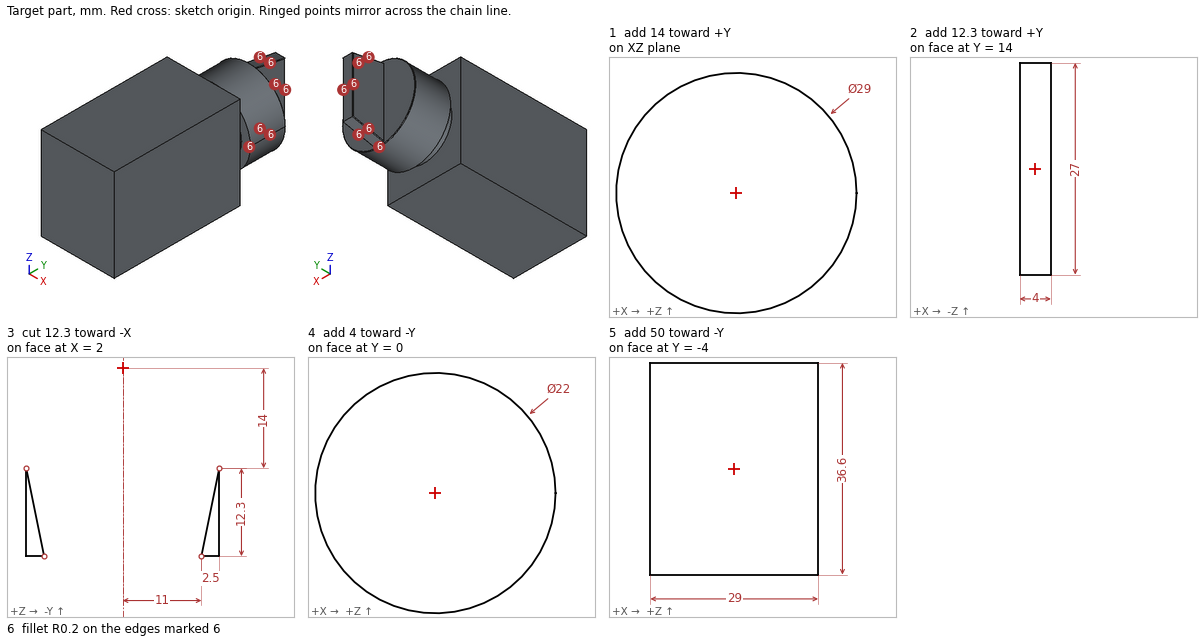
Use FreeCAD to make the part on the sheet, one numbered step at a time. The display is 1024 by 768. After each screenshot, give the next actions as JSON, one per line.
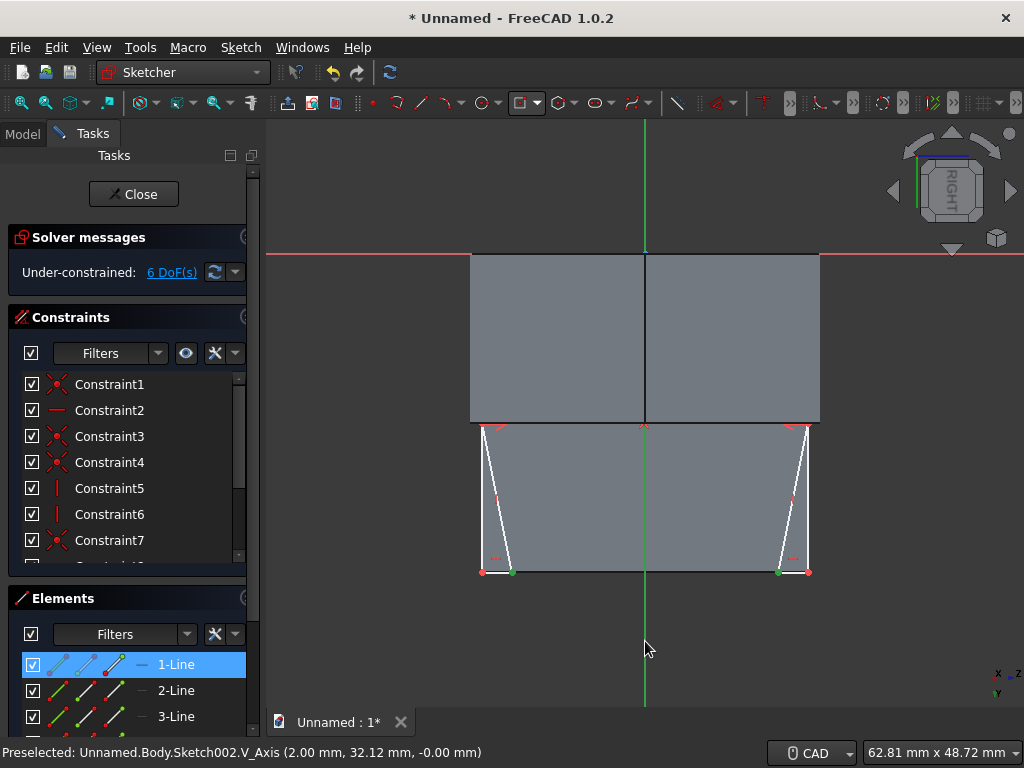
{"action": "key", "text": "s"}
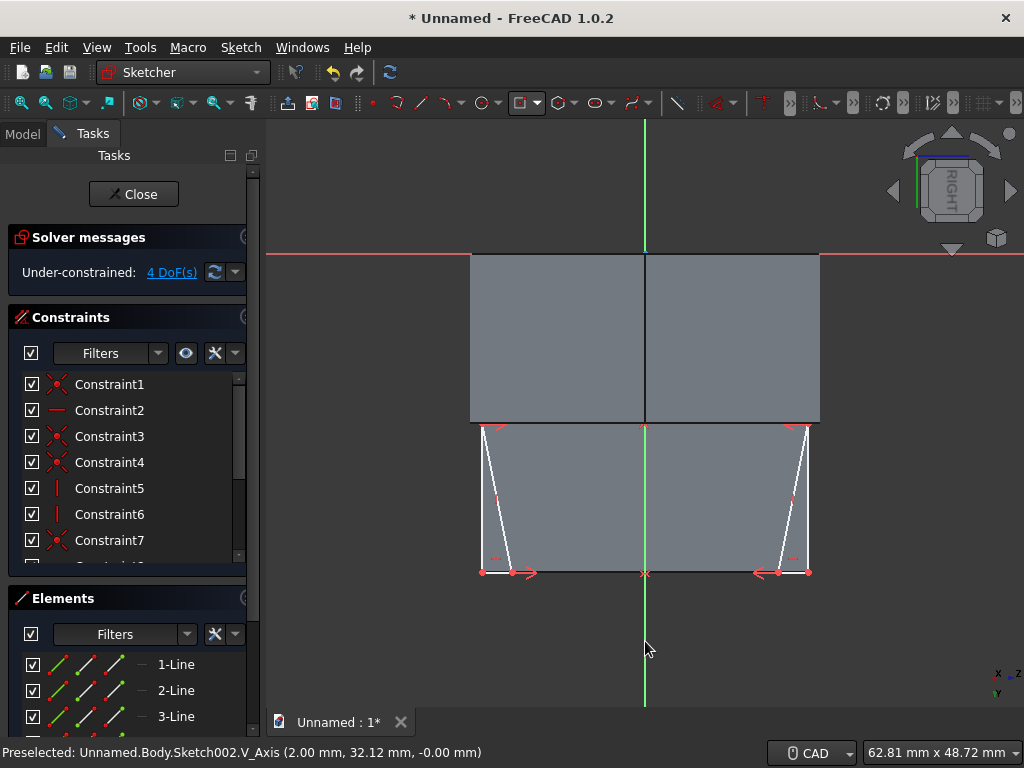
{"action": "left_click", "coordinate": [716, 104]}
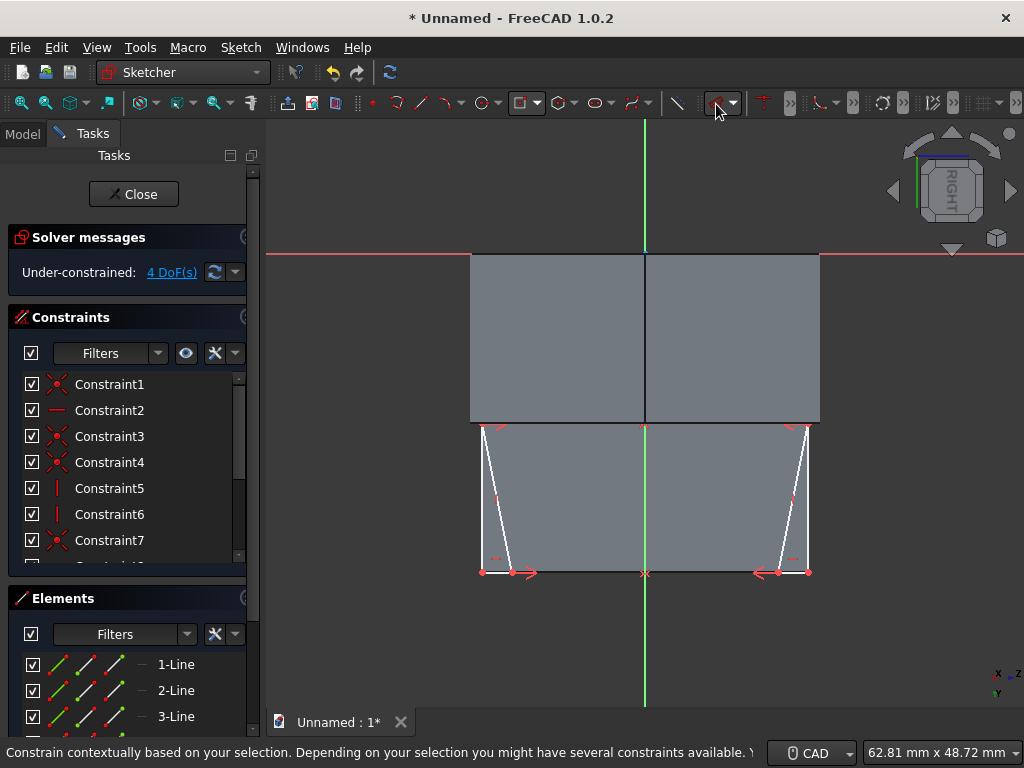
{"action": "scroll", "coordinate": [790, 573], "scroll_direction": "up", "scroll_amount": 2}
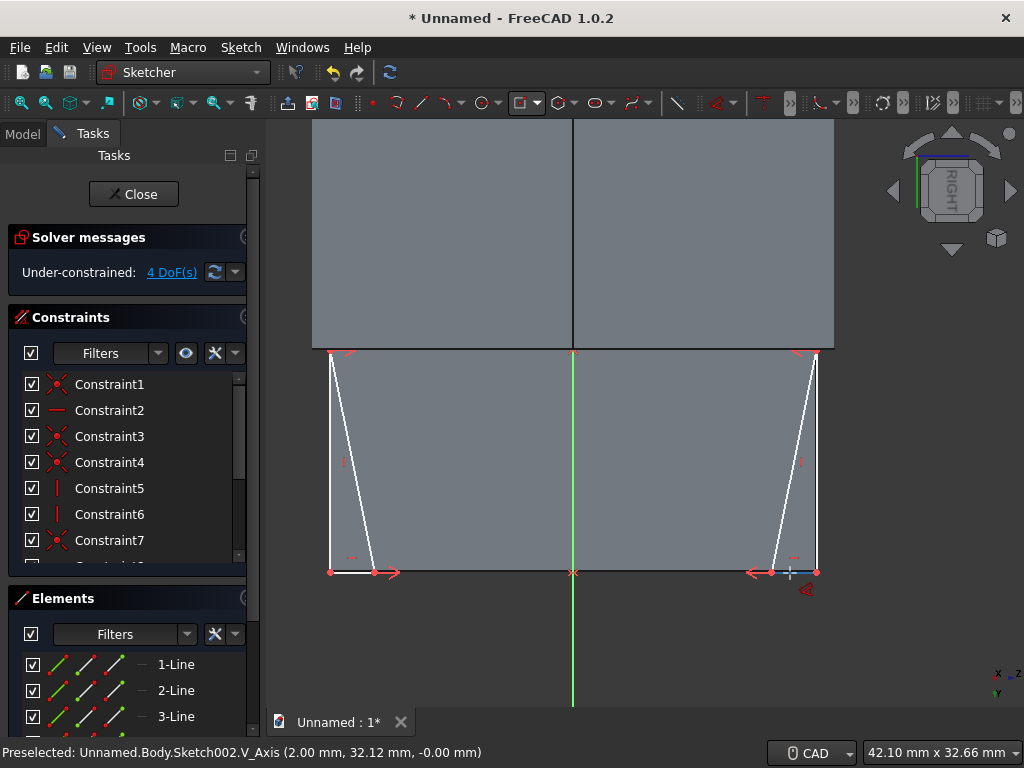
{"action": "left_click", "coordinate": [790, 573]}
{"action": "left_click", "coordinate": [794, 607]}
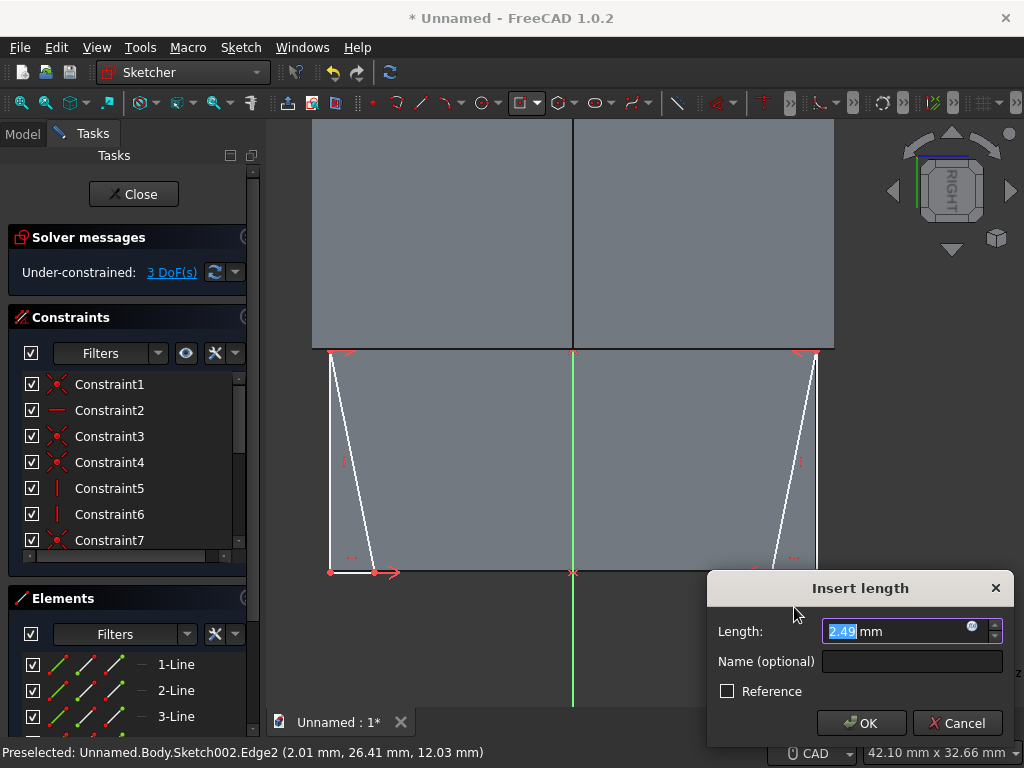
{"action": "type", "text": "2.5"}
{"action": "key", "text": "Return"}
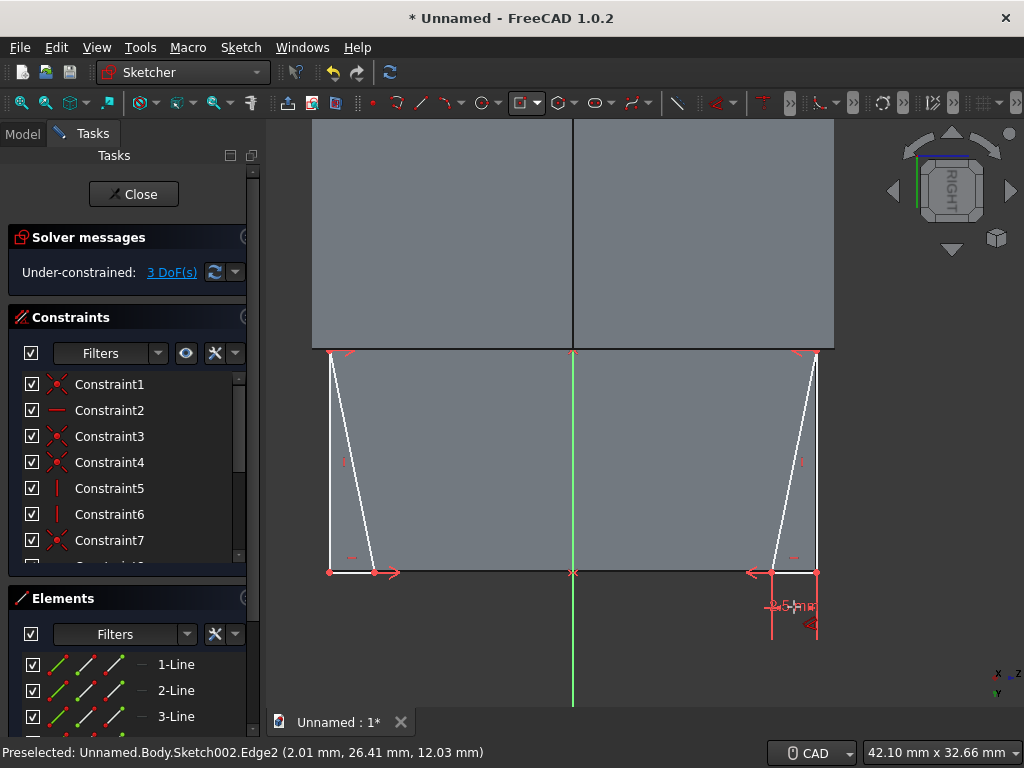
{"action": "left_click", "coordinate": [817, 350]}
{"action": "left_click", "coordinate": [851, 249]}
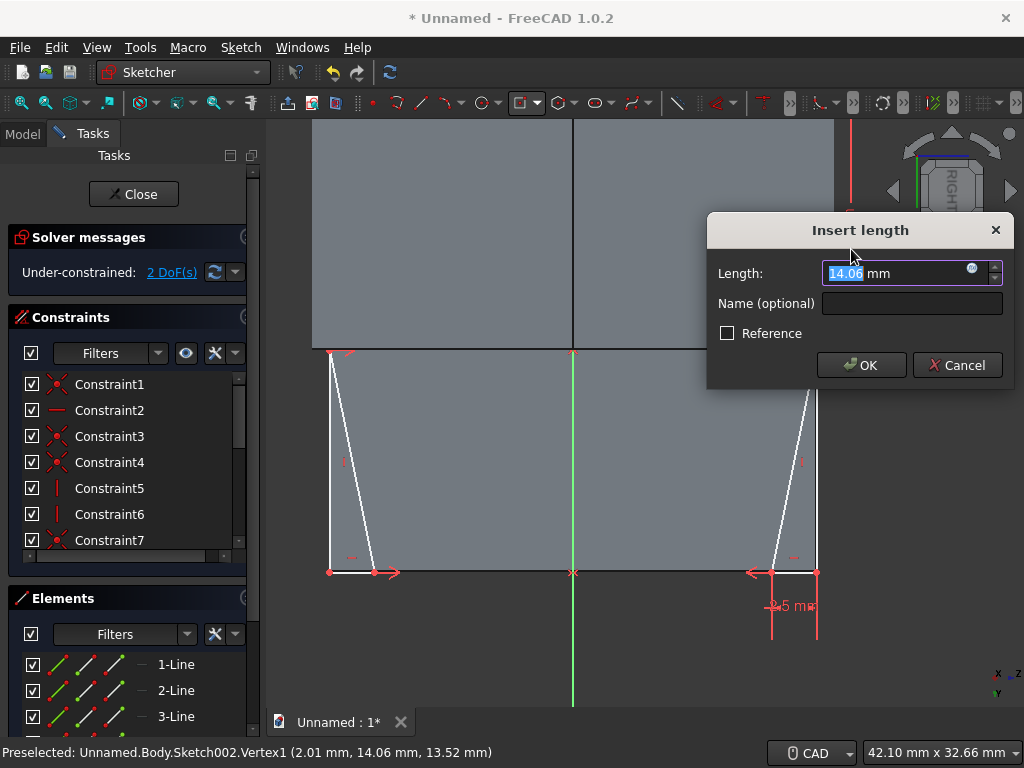
{"action": "type", "text": "14"}
{"action": "key", "text": "Return"}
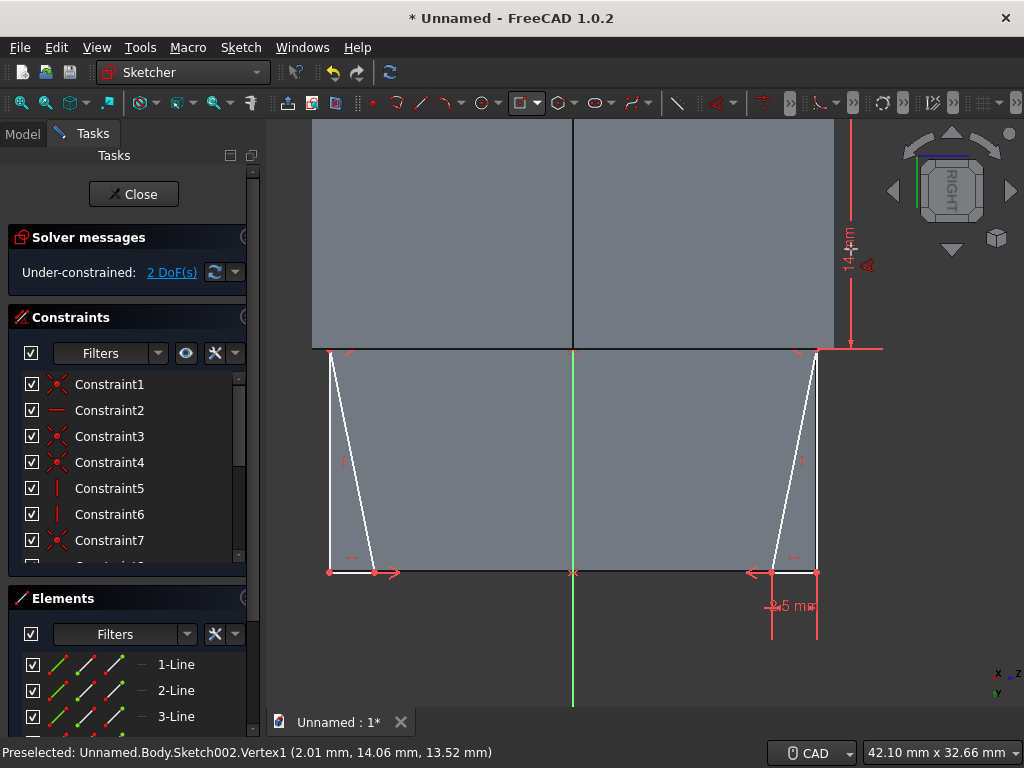
{"action": "left_click", "coordinate": [772, 573]}
{"action": "left_click", "coordinate": [673, 607]}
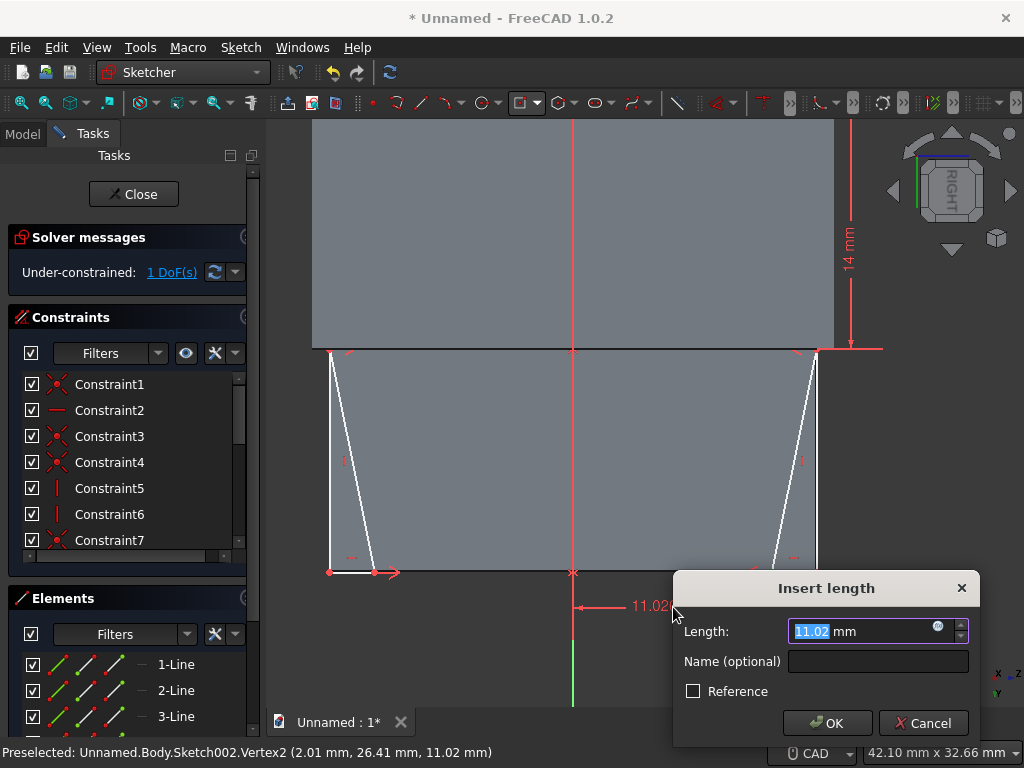
{"action": "type", "text": "11"}
{"action": "key", "text": "Return"}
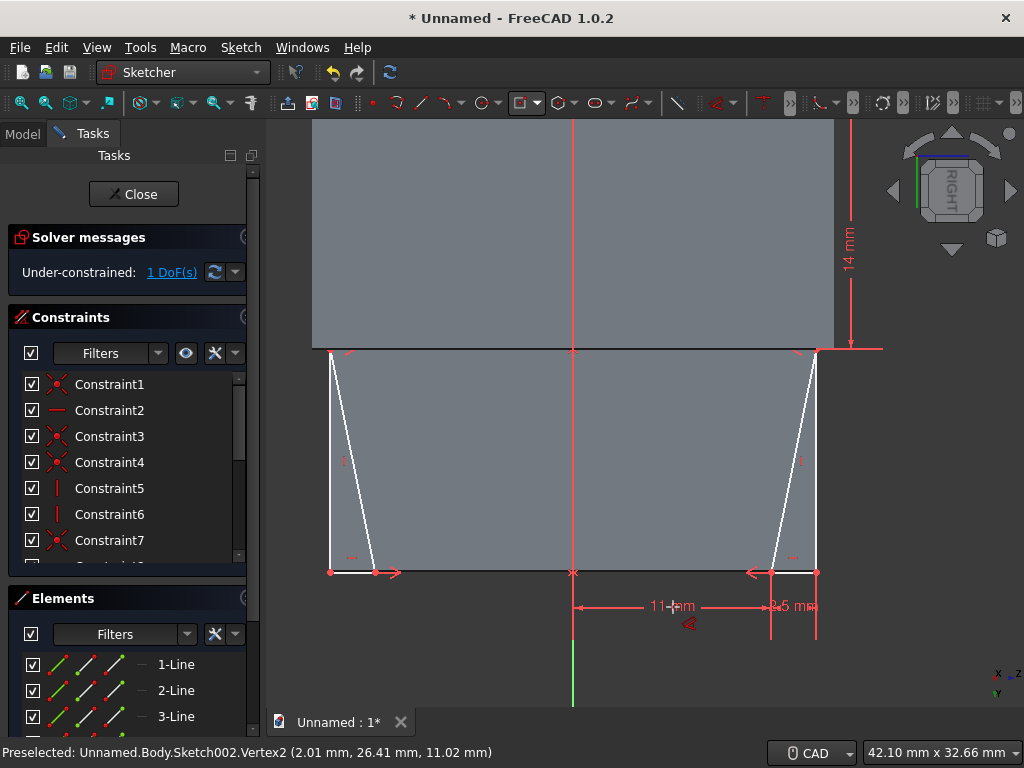
{"action": "left_click", "coordinate": [816, 506]}
{"action": "left_click", "coordinate": [850, 461]}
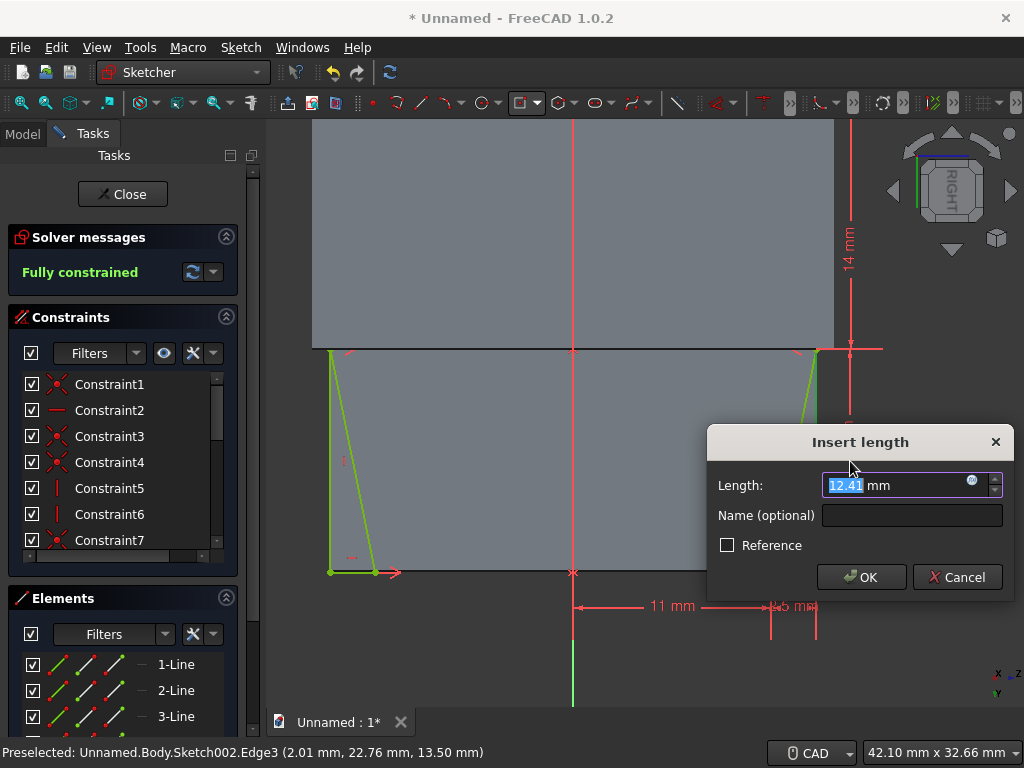
{"action": "type", "text": "12.3"}
{"action": "key", "text": "Return"}
{"action": "key", "text": "Escape"}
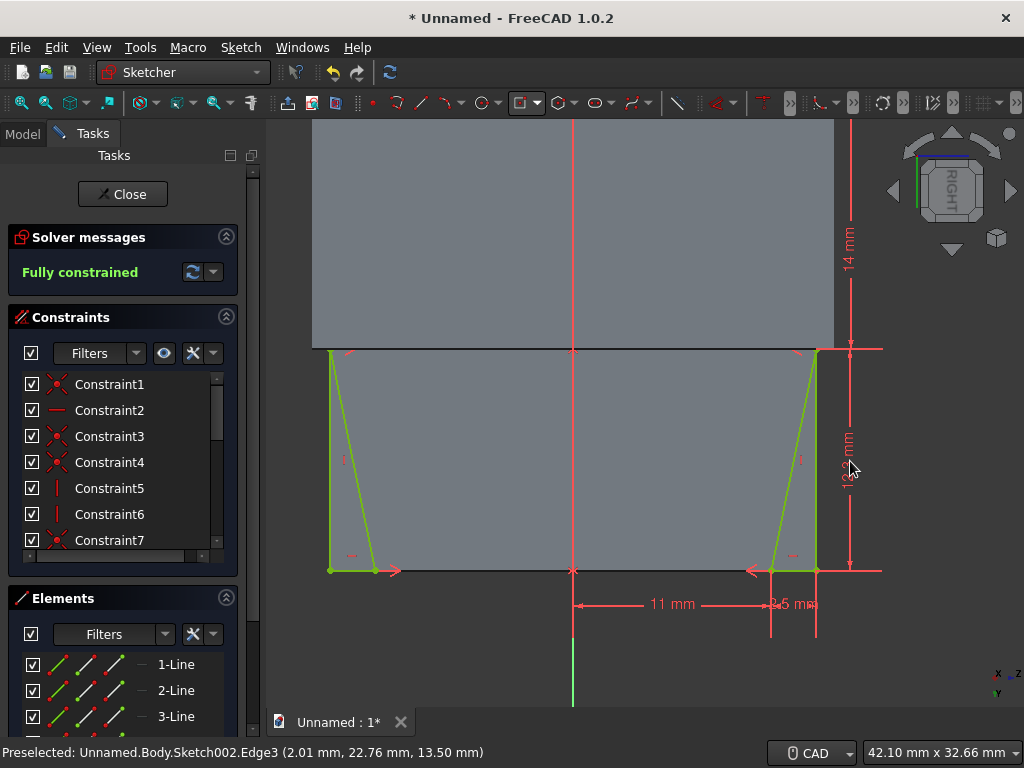
{"action": "left_click", "coordinate": [123, 194]}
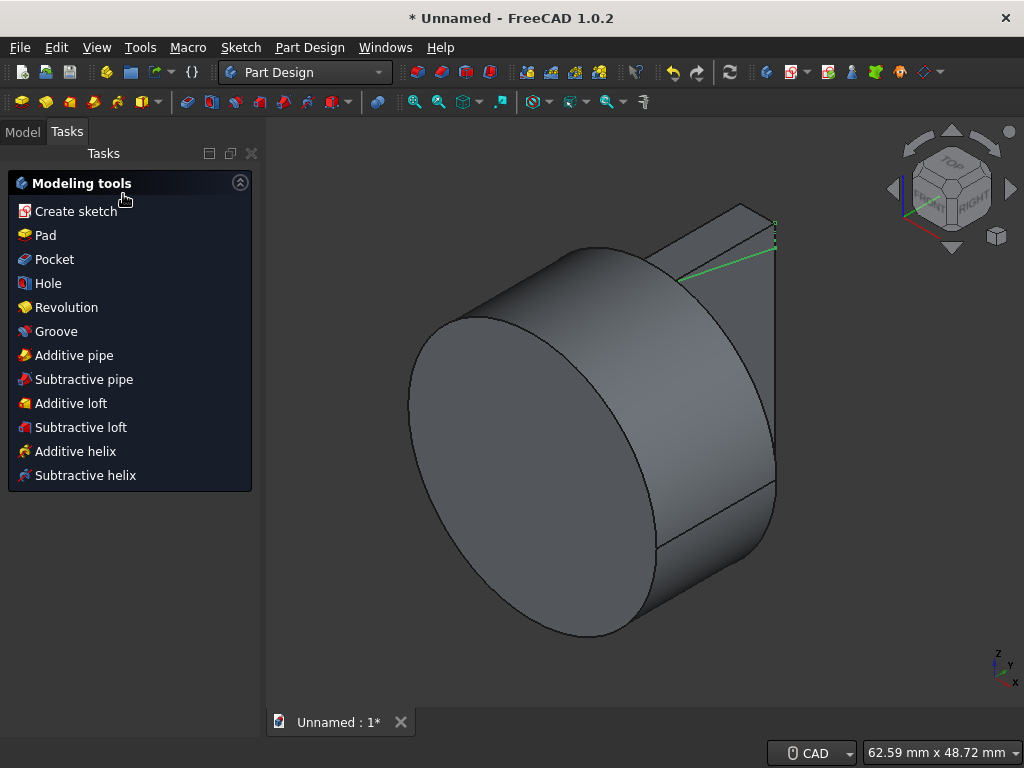
{"action": "left_click", "coordinate": [188, 102]}